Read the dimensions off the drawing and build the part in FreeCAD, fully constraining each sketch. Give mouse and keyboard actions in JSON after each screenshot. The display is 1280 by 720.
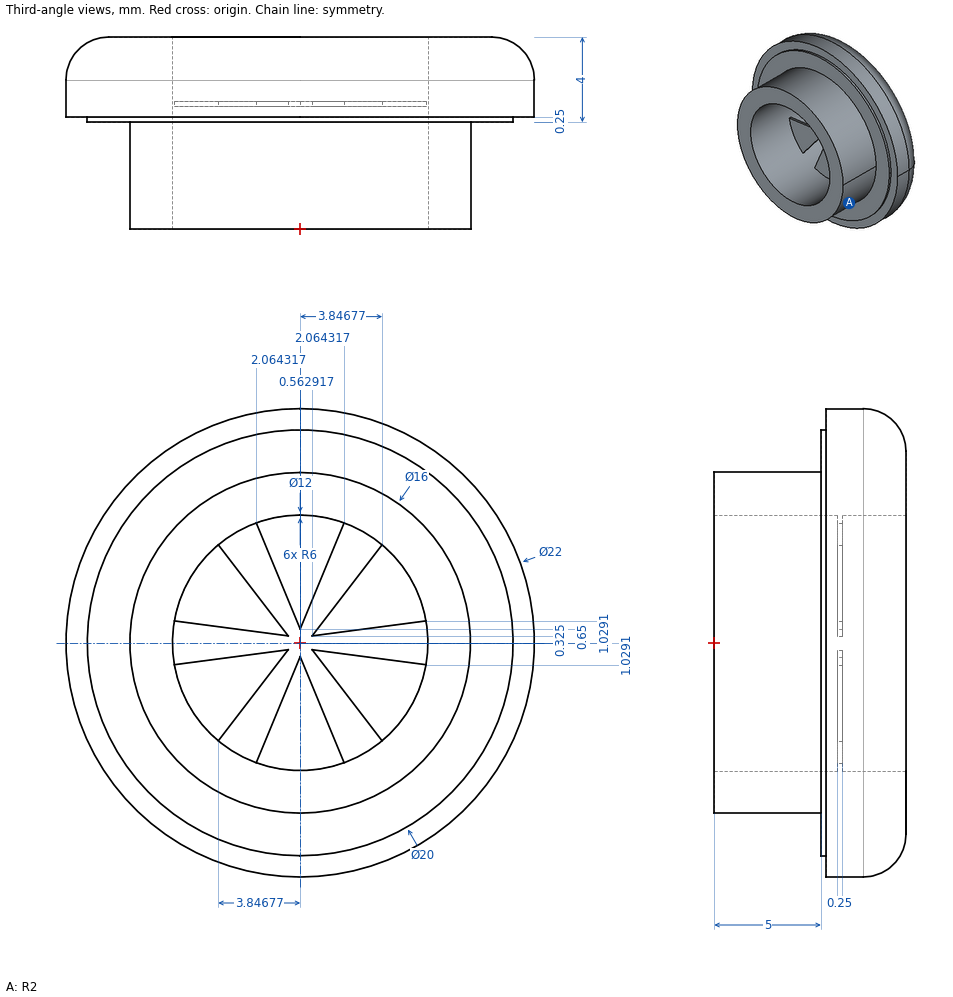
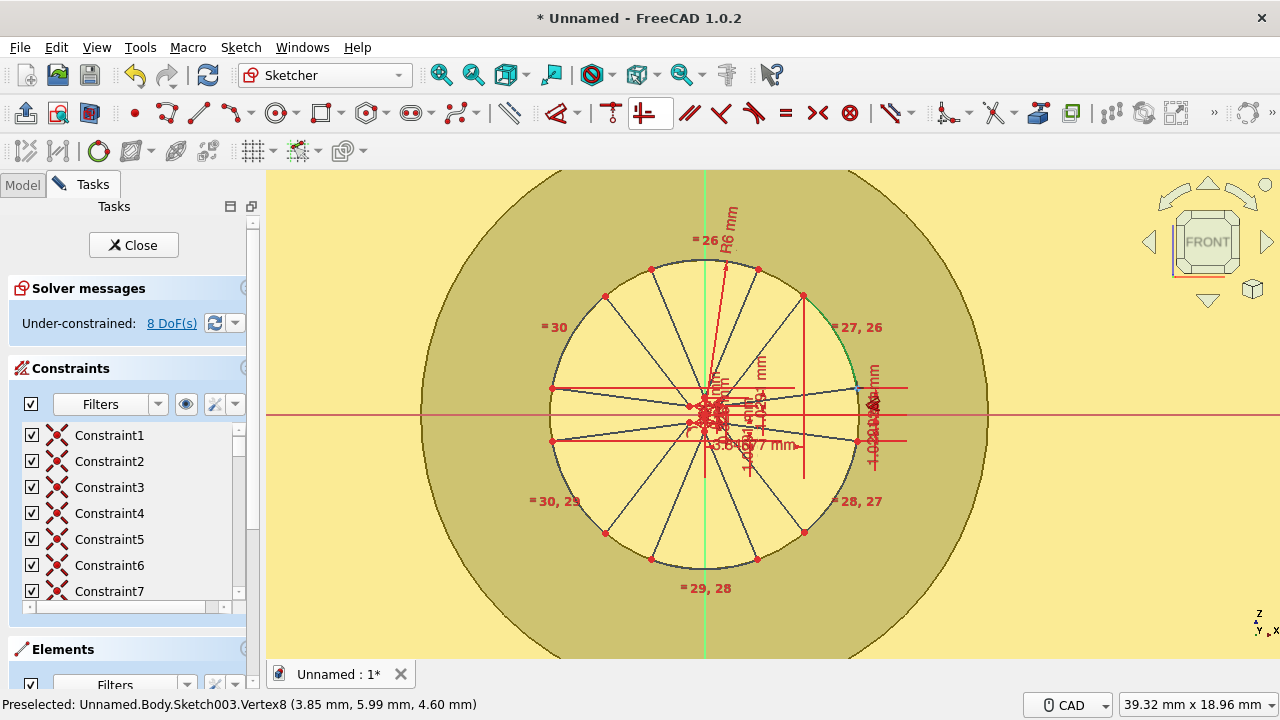
{"action": "left_click", "coordinate": [804, 533]}
{"action": "left_click", "coordinate": [777, 567]}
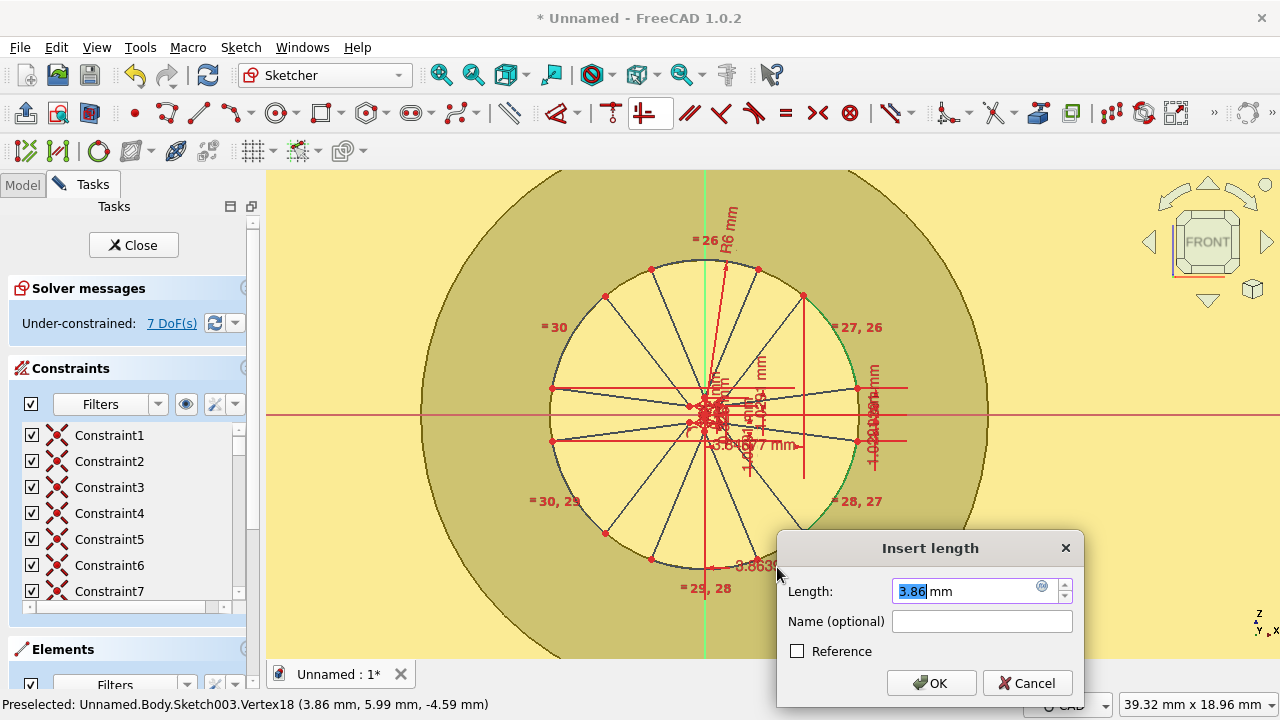
{"action": "type", "text": "3.84677"}
{"action": "key", "text": "Return"}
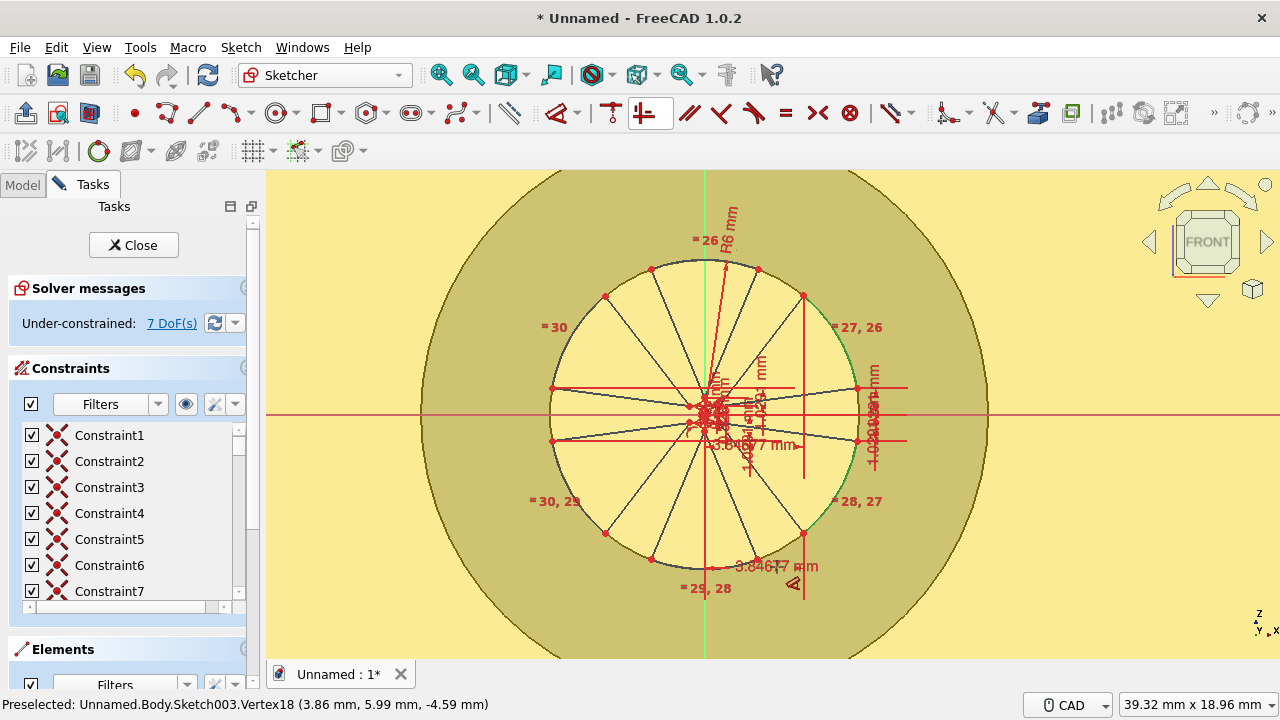
{"action": "left_click", "coordinate": [606, 533]}
{"action": "left_click", "coordinate": [632, 567]}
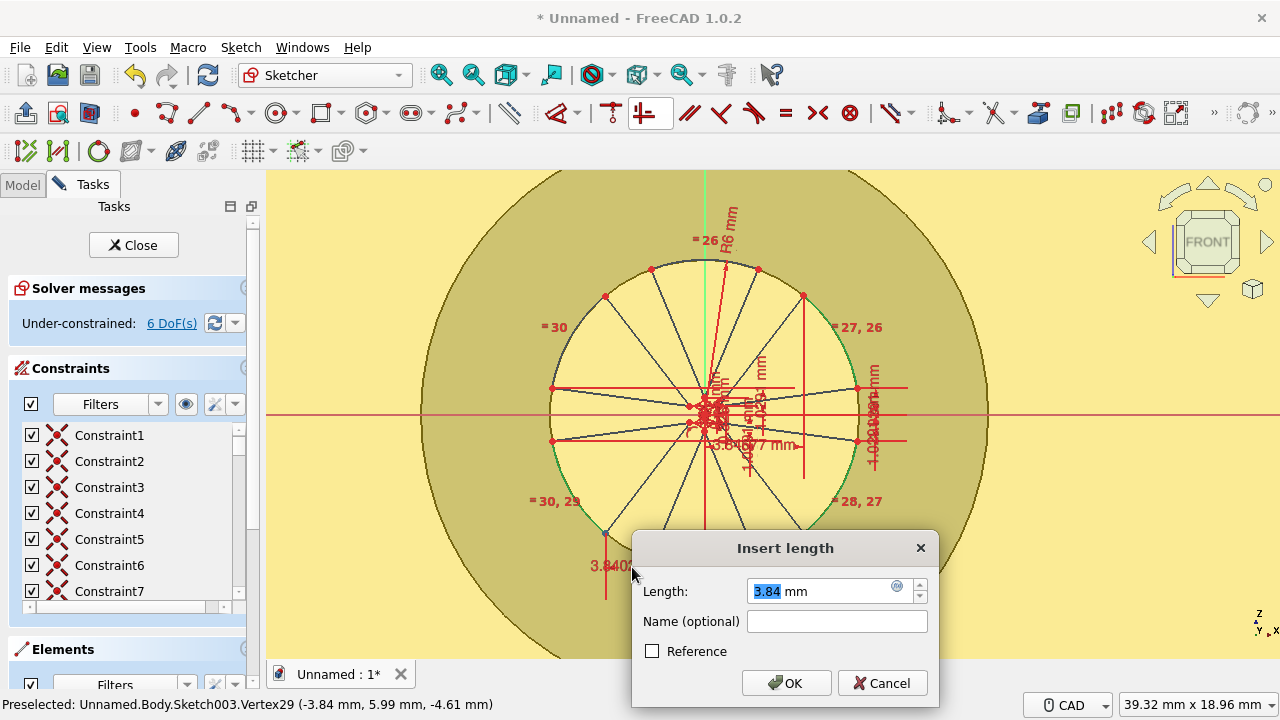
{"action": "type", "text": "3.84677"}
{"action": "key", "text": "Return"}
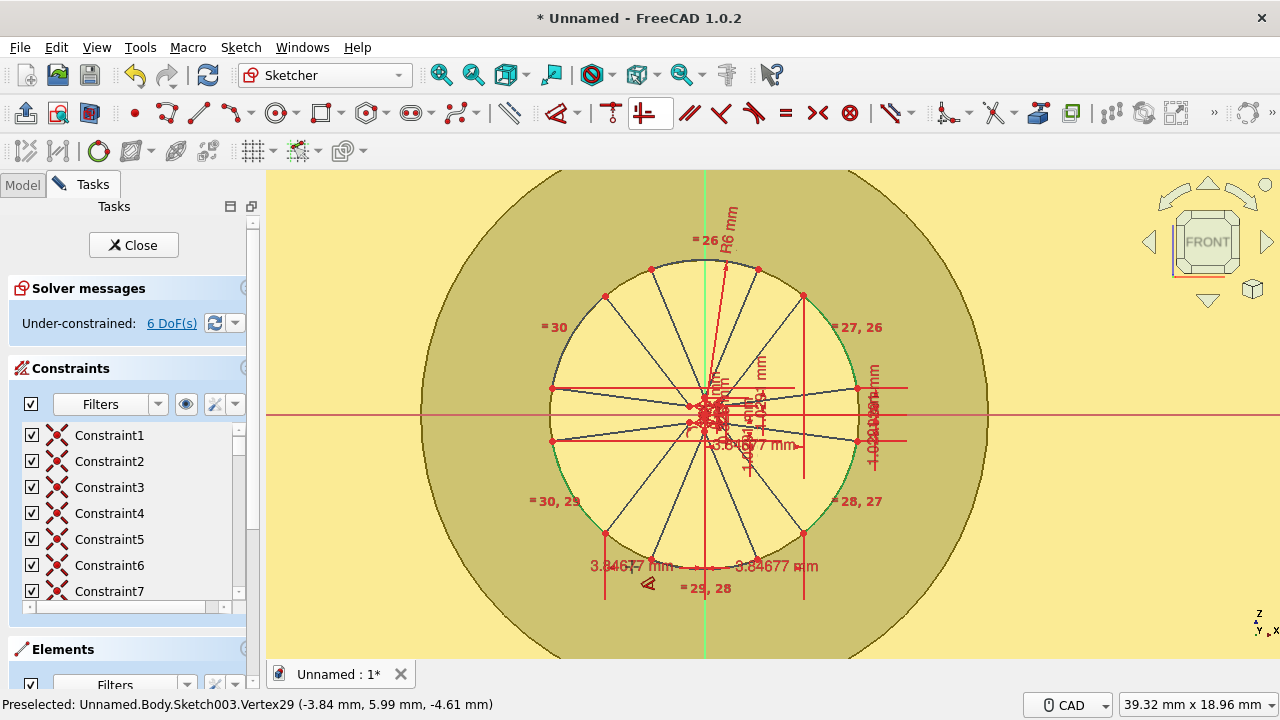
{"action": "left_click", "coordinate": [605, 296]}
{"action": "left_click", "coordinate": [632, 262]}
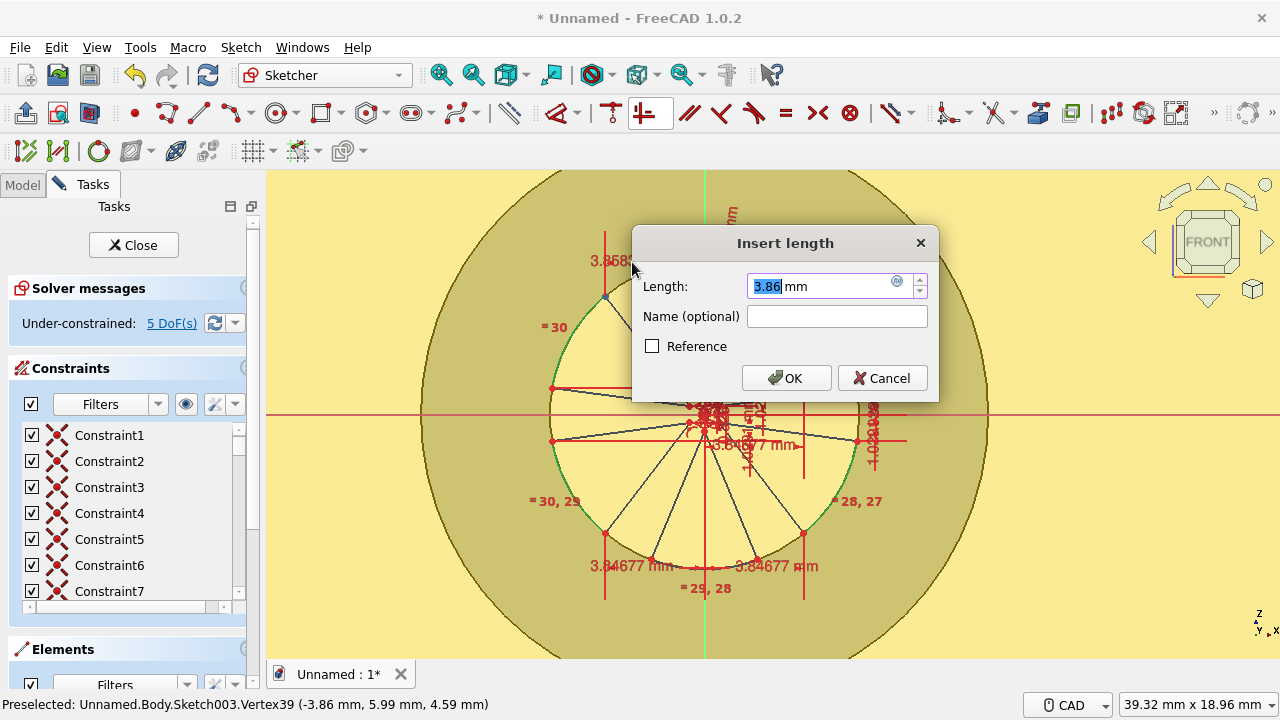
{"action": "type", "text": "3.84677"}
{"action": "key", "text": "Return"}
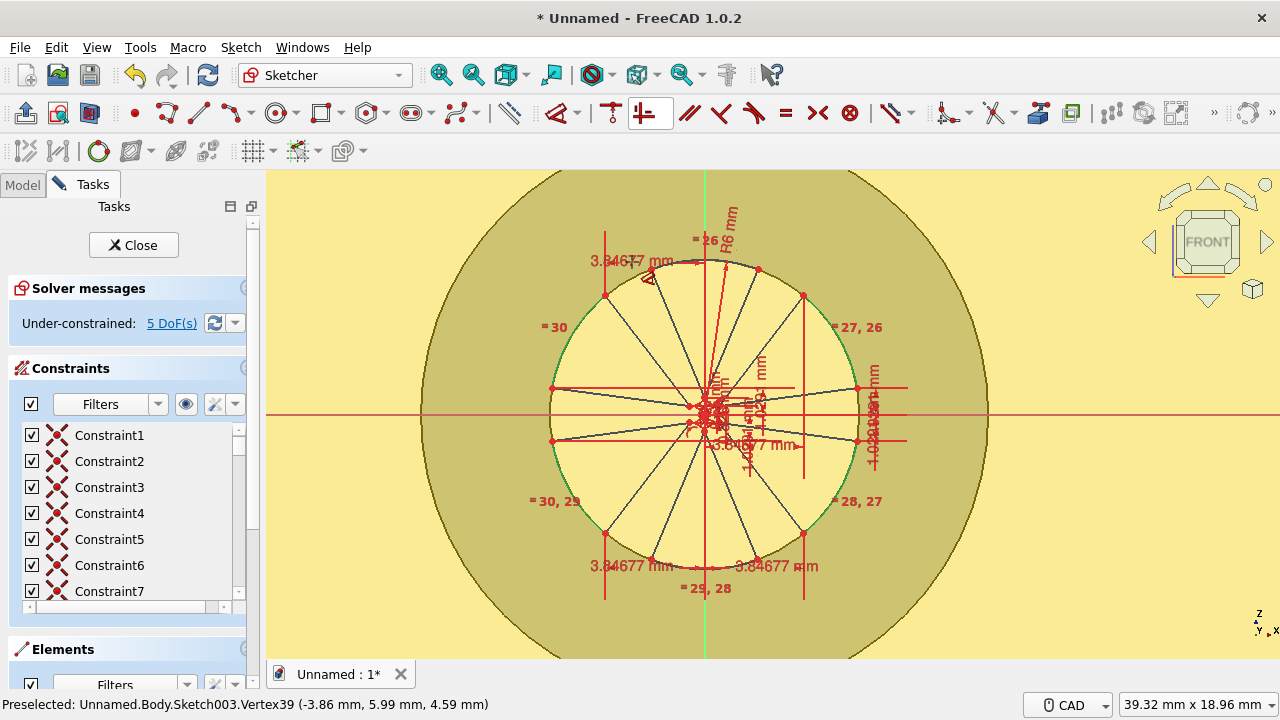
{"action": "left_click", "coordinate": [651, 269]}
{"action": "left_click", "coordinate": [659, 235]}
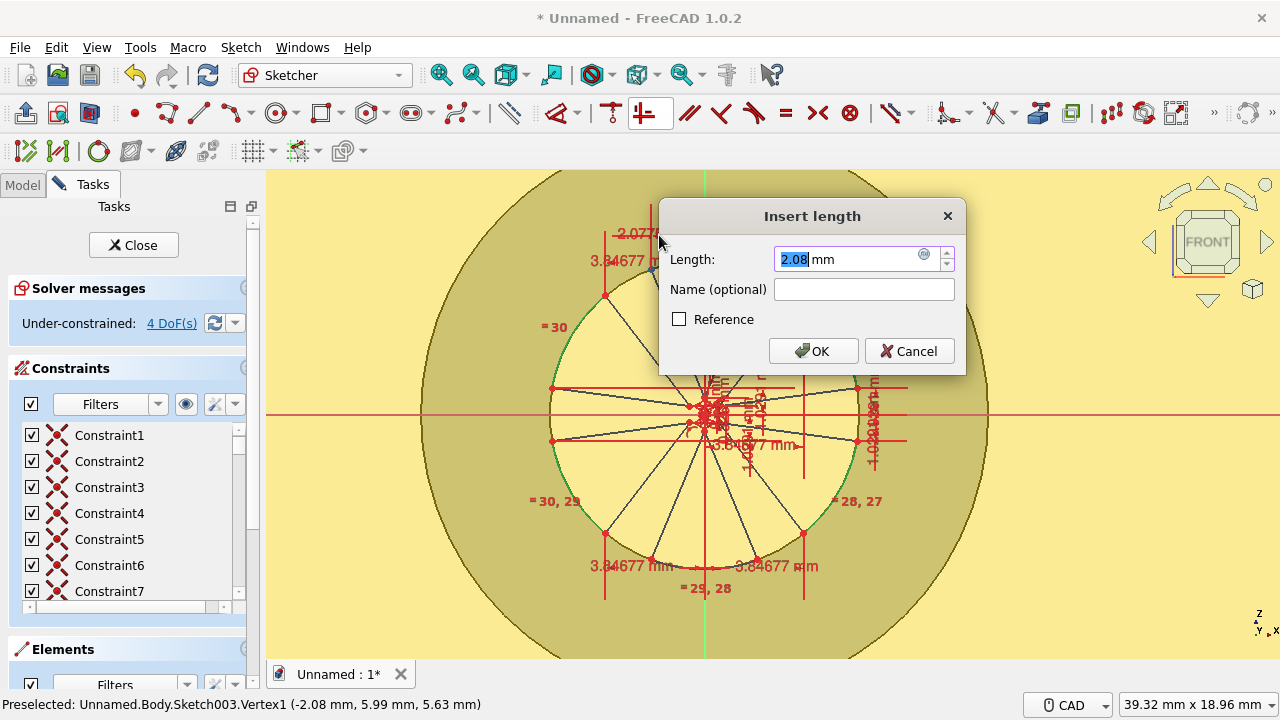
{"action": "type", "text": "2.064317"}
{"action": "key", "text": "Return"}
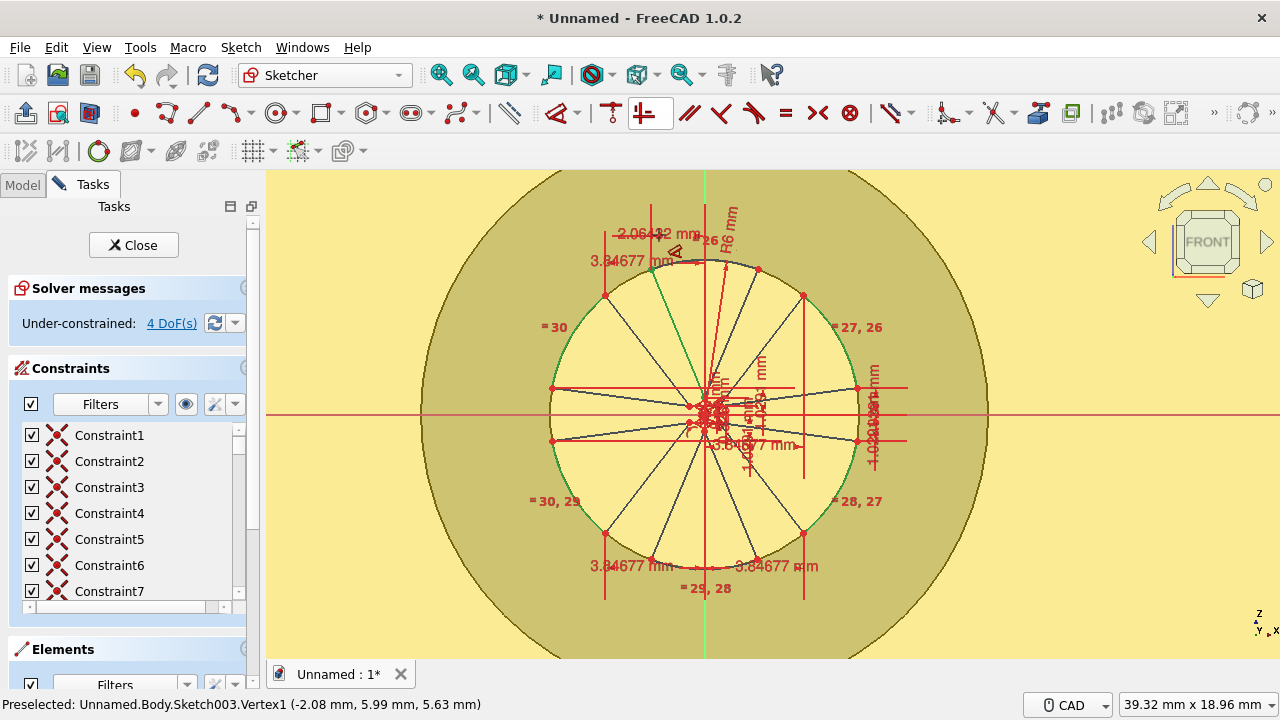
{"action": "left_click", "coordinate": [758, 269]}
{"action": "left_click", "coordinate": [731, 211]}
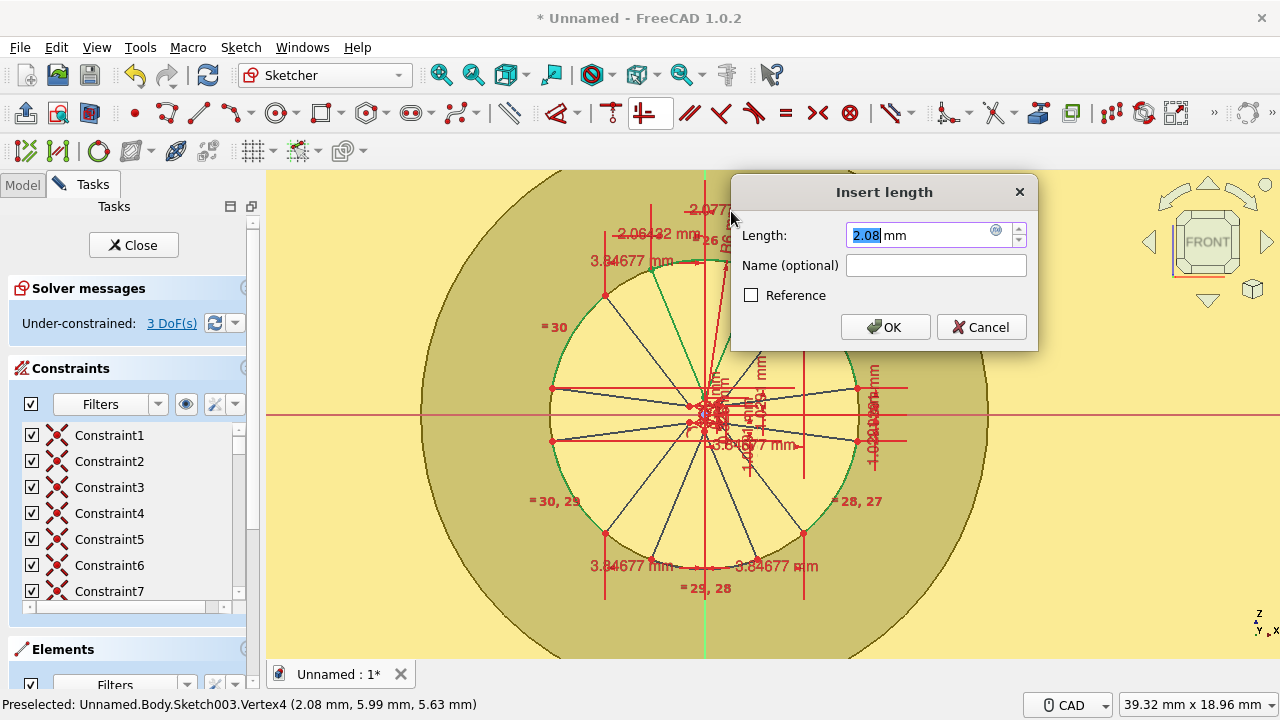
{"action": "type", "text": "2.064317"}
{"action": "key", "text": "Return"}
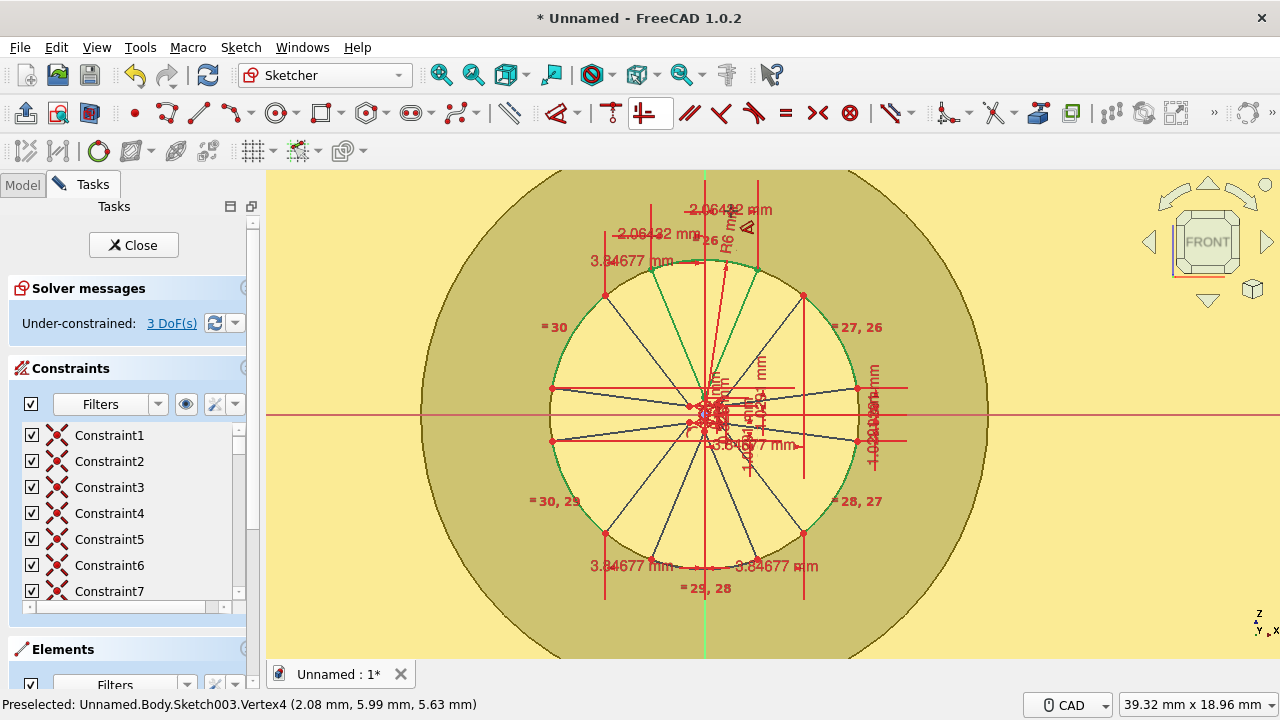
{"action": "scroll", "coordinate": [719, 406], "scroll_direction": "up", "scroll_amount": 6}